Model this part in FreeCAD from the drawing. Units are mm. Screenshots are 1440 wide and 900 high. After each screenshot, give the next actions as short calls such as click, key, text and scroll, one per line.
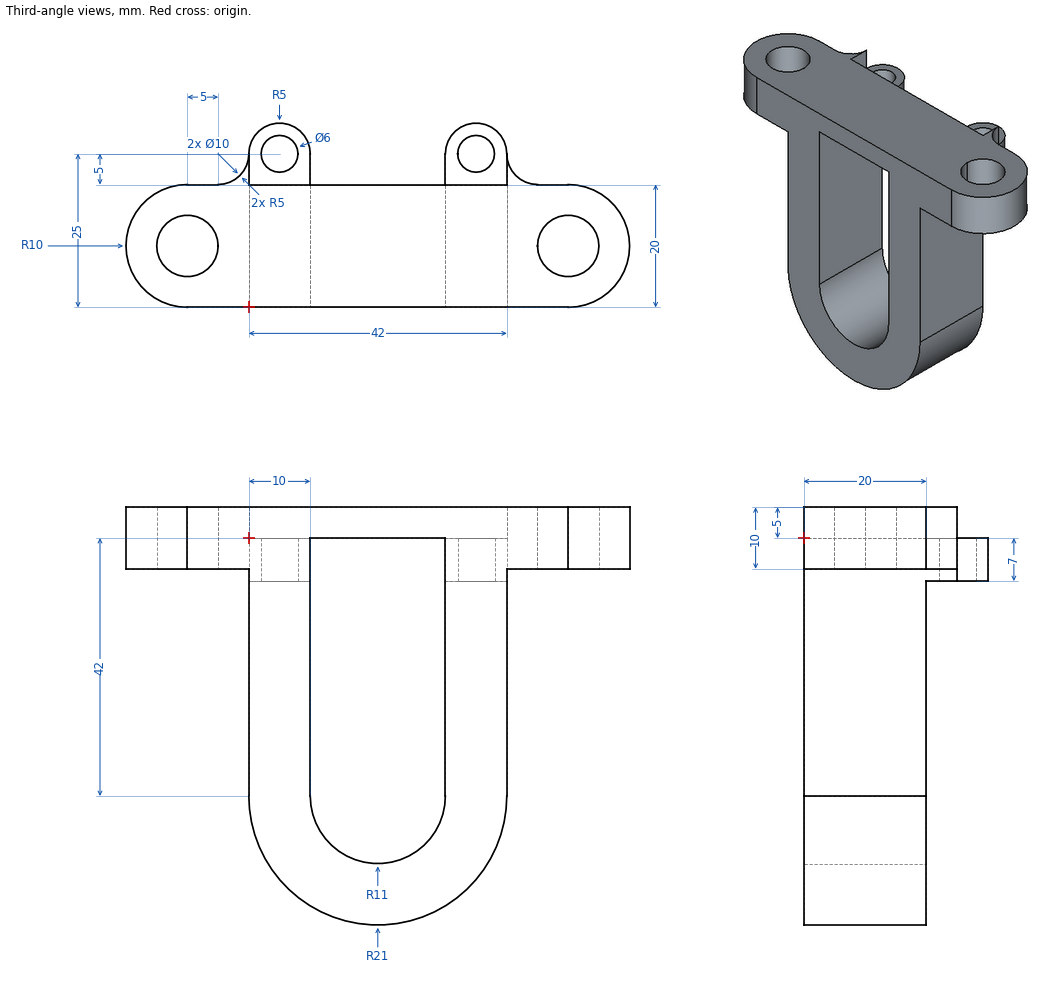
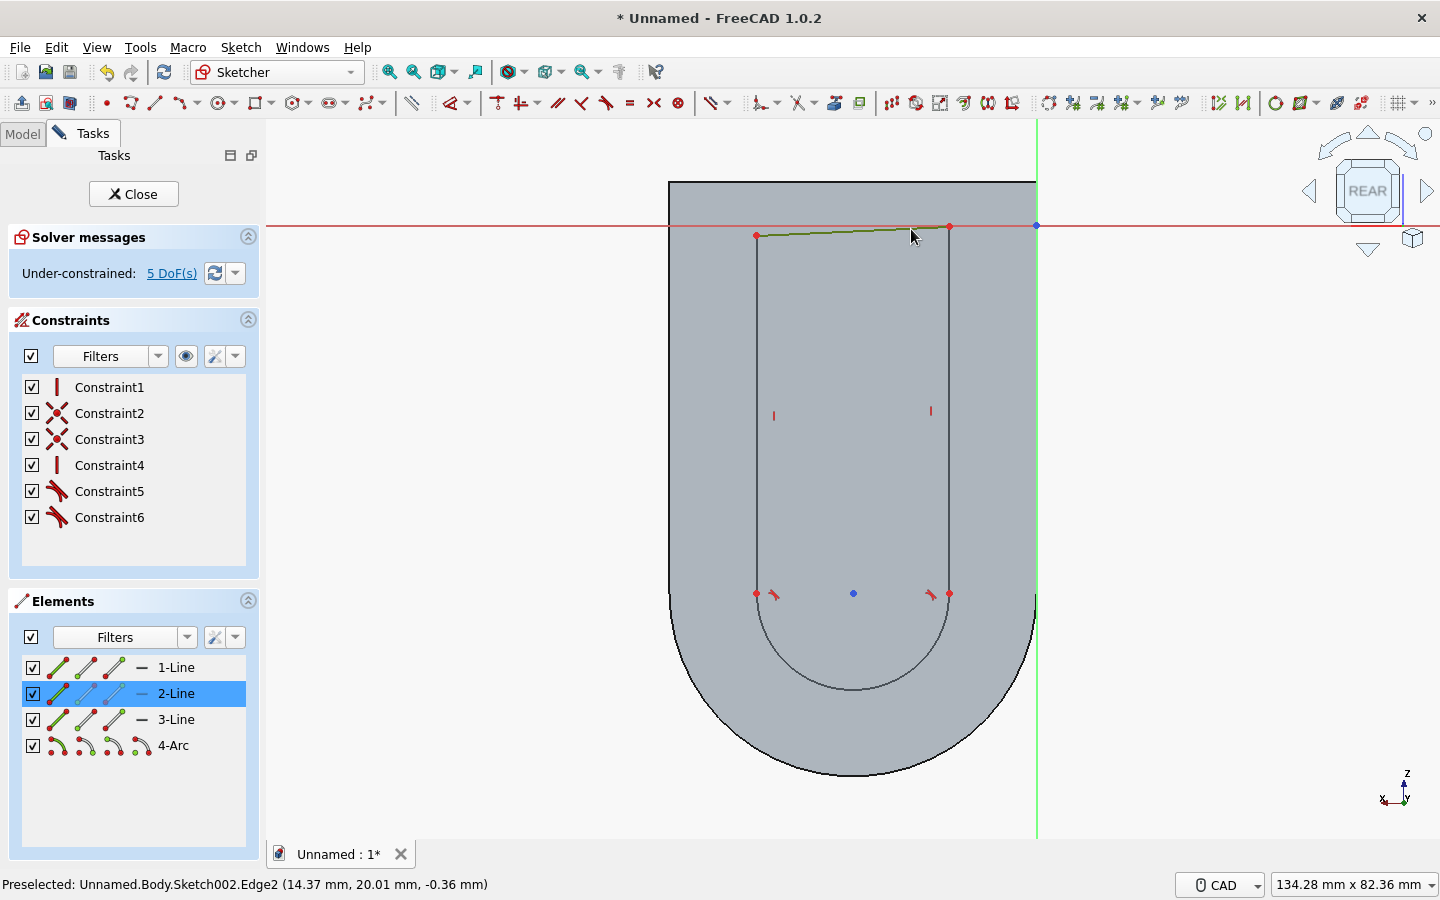
click(540, 104)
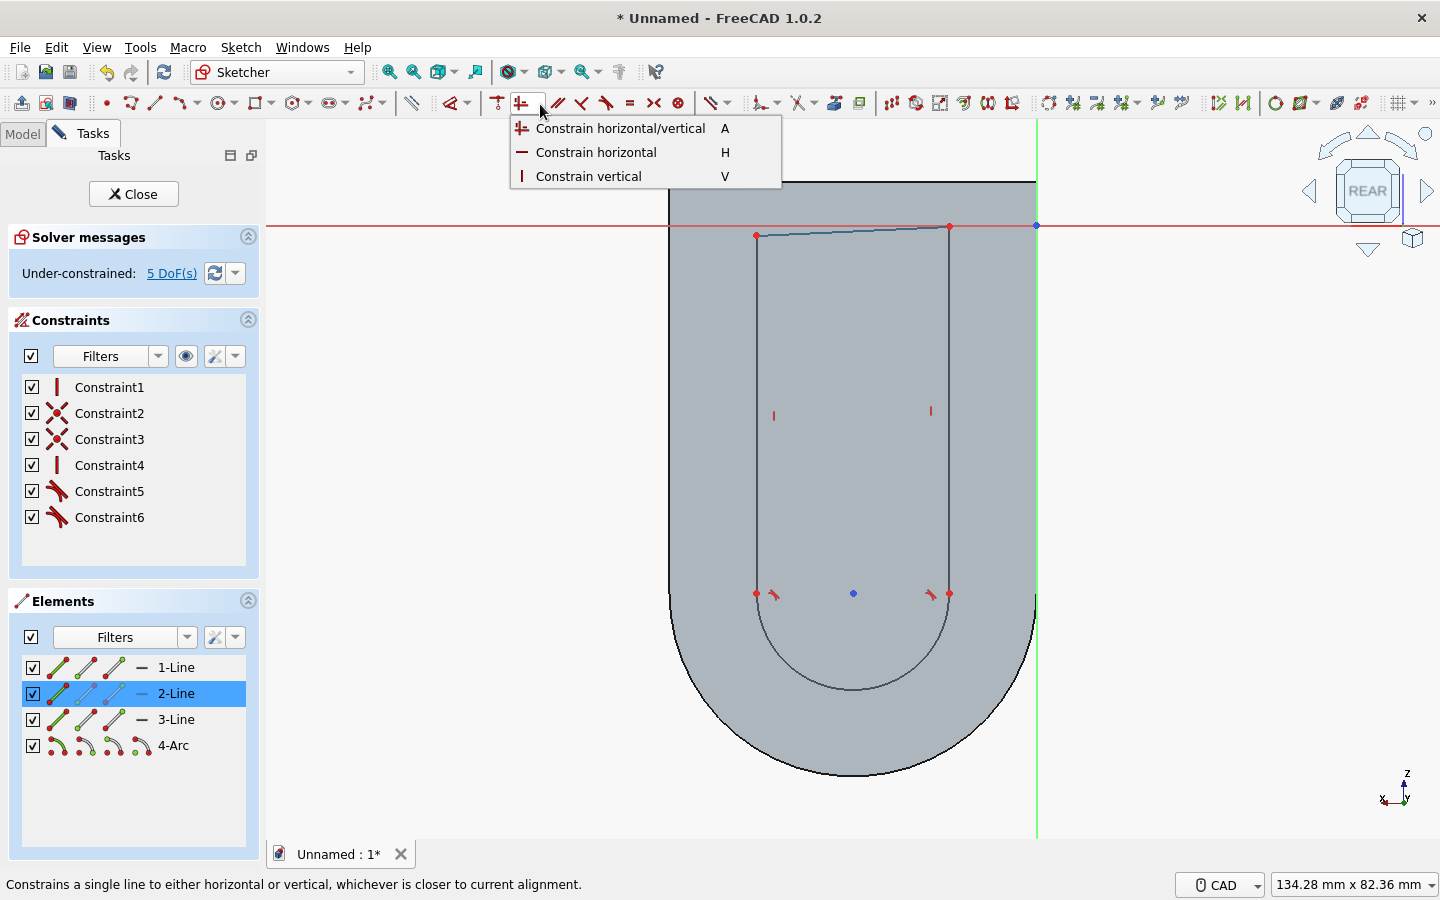
click(646, 152)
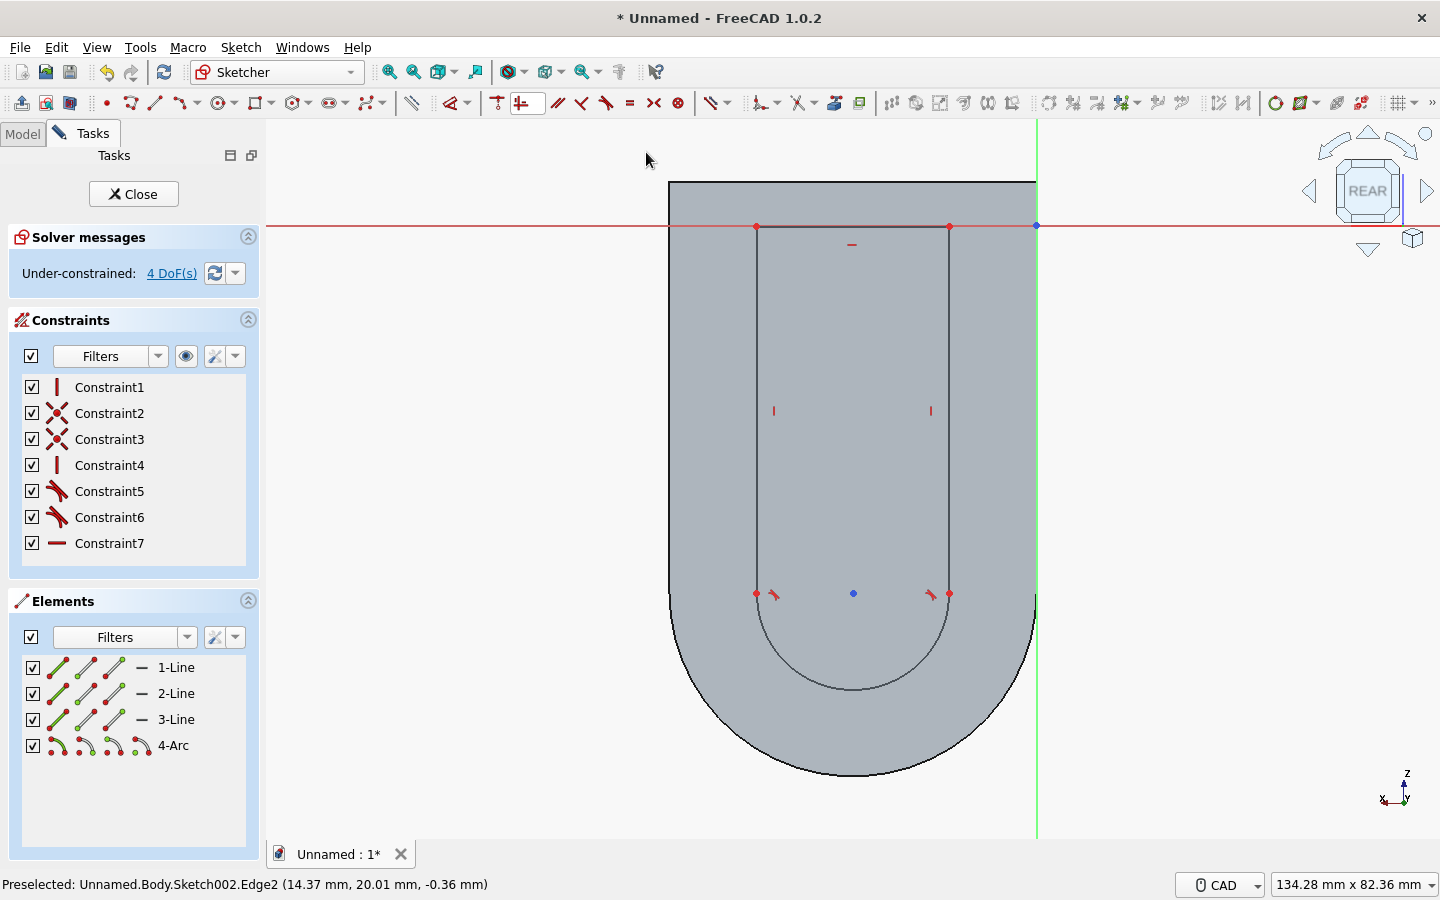
click(450, 104)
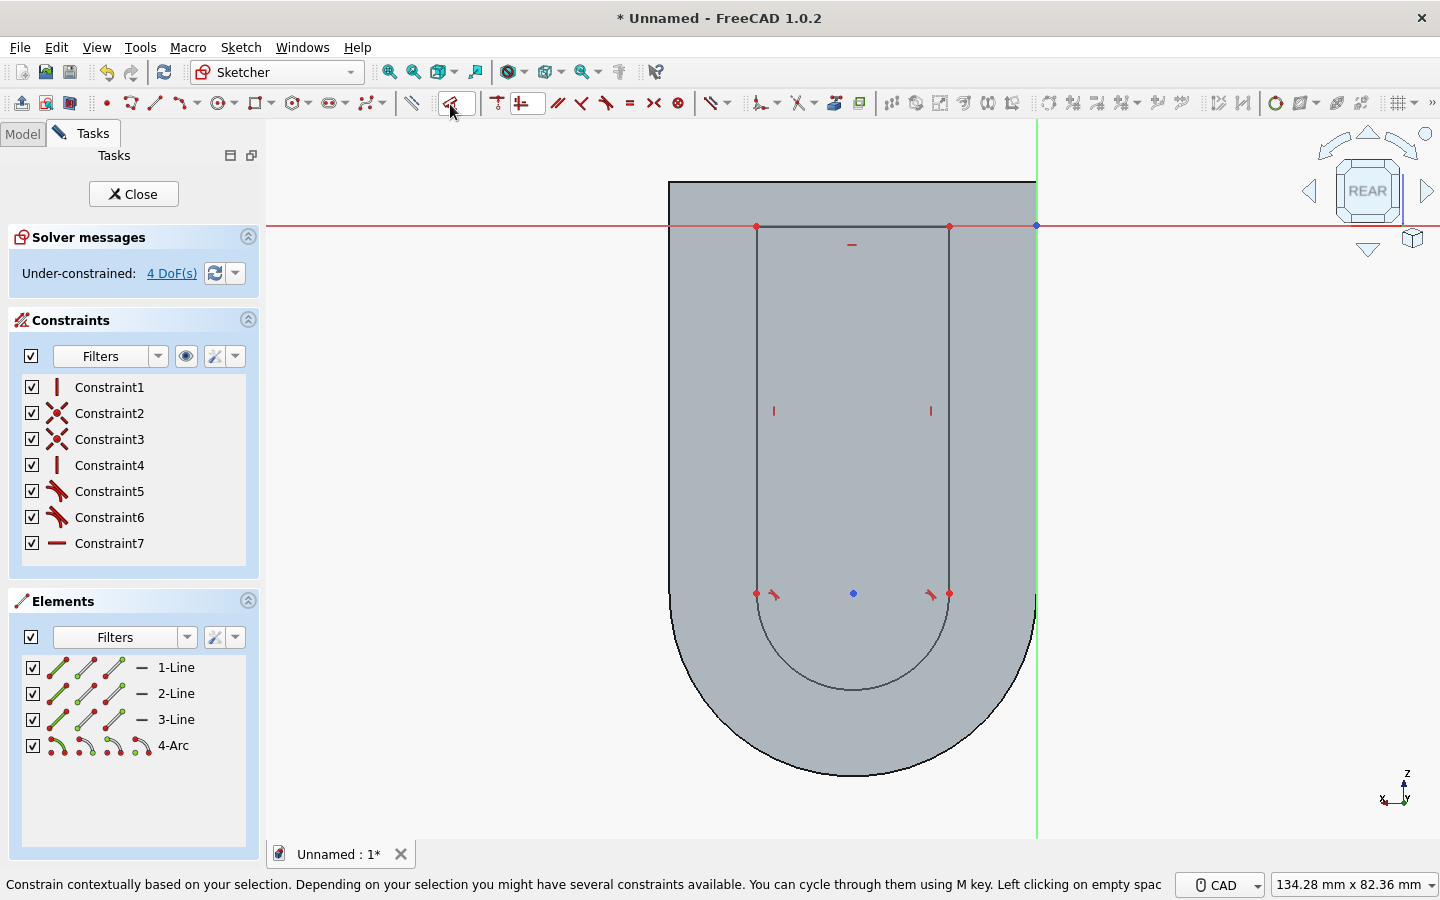
click(797, 672)
click(778, 698)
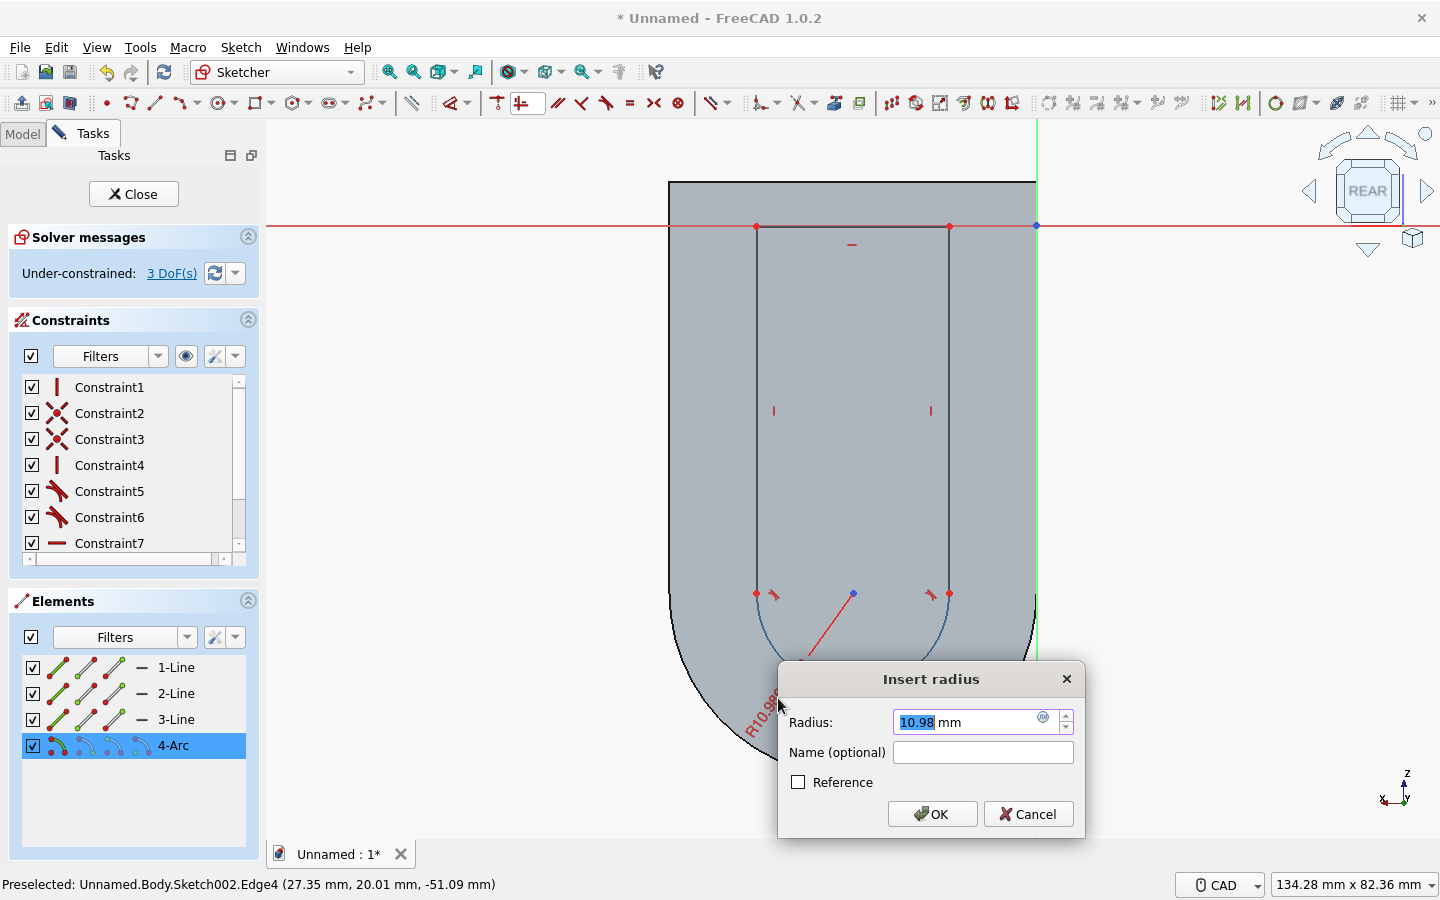
text(11)
key(Return)
key(Escape)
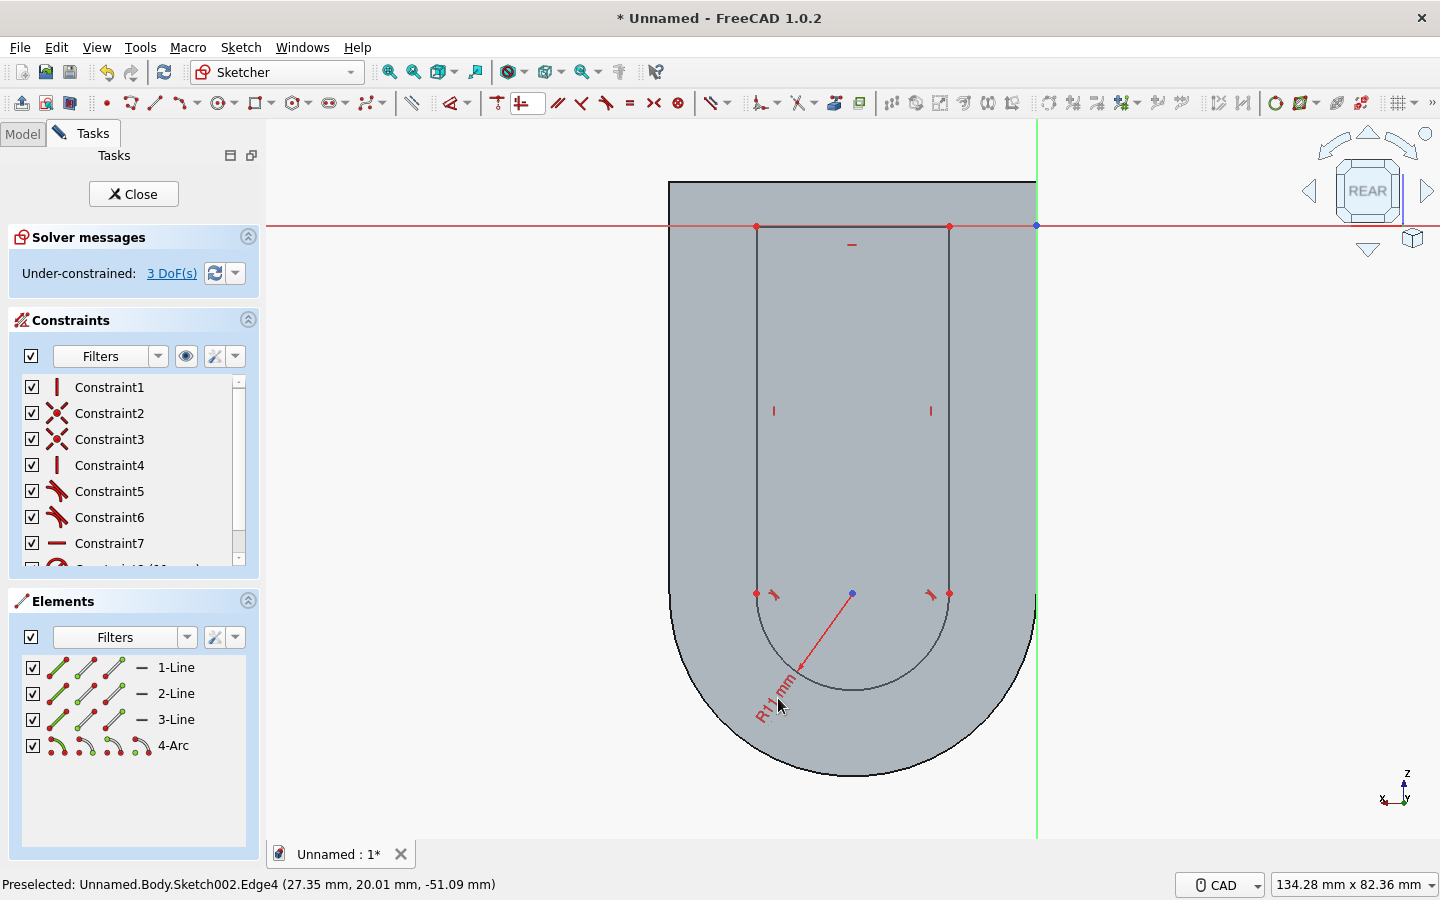
click(949, 227)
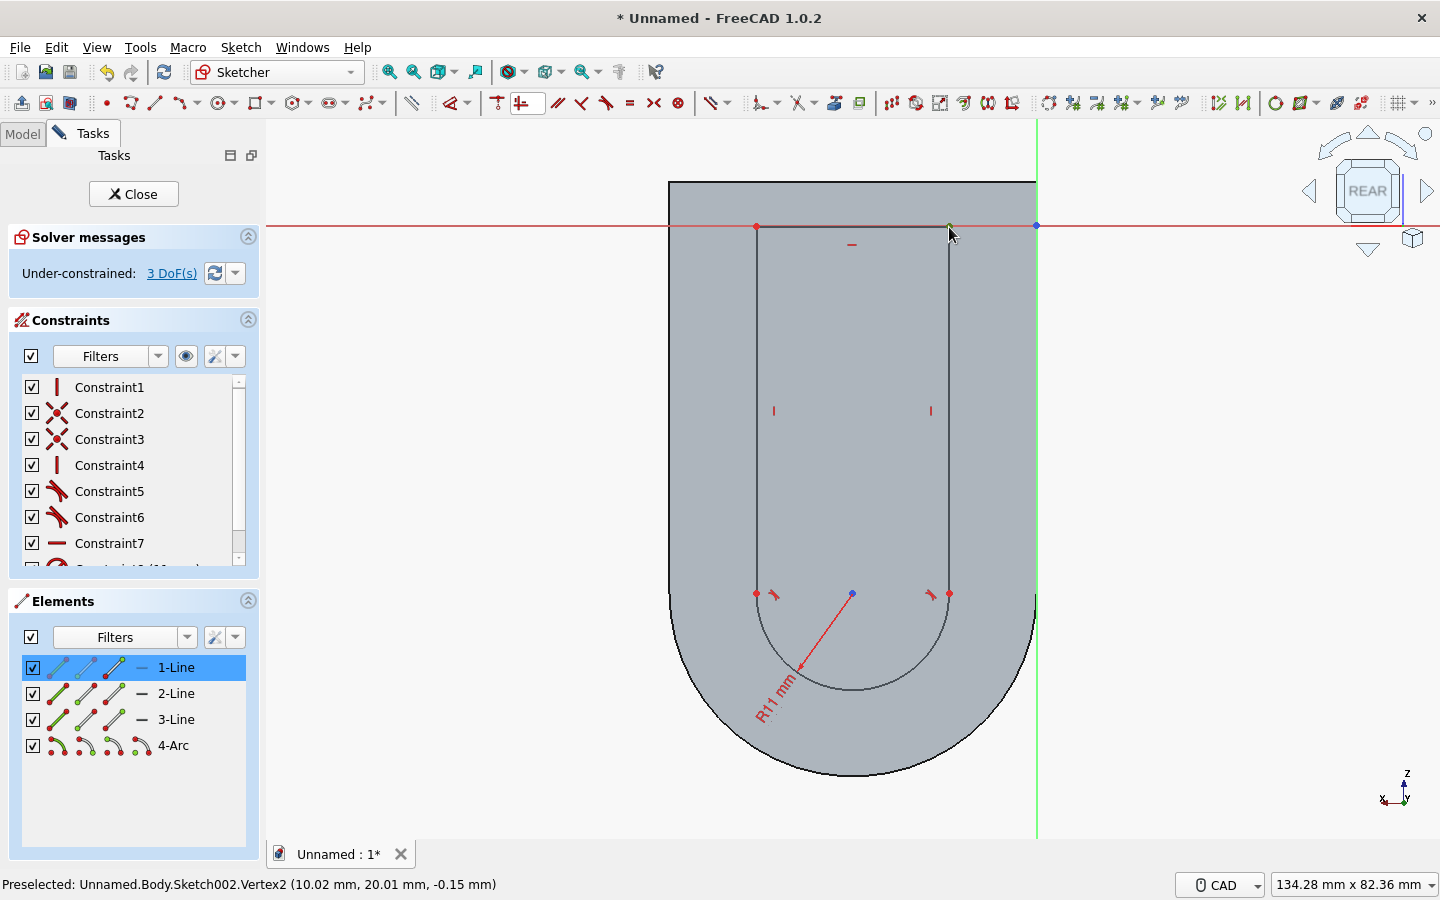
click(364, 226)